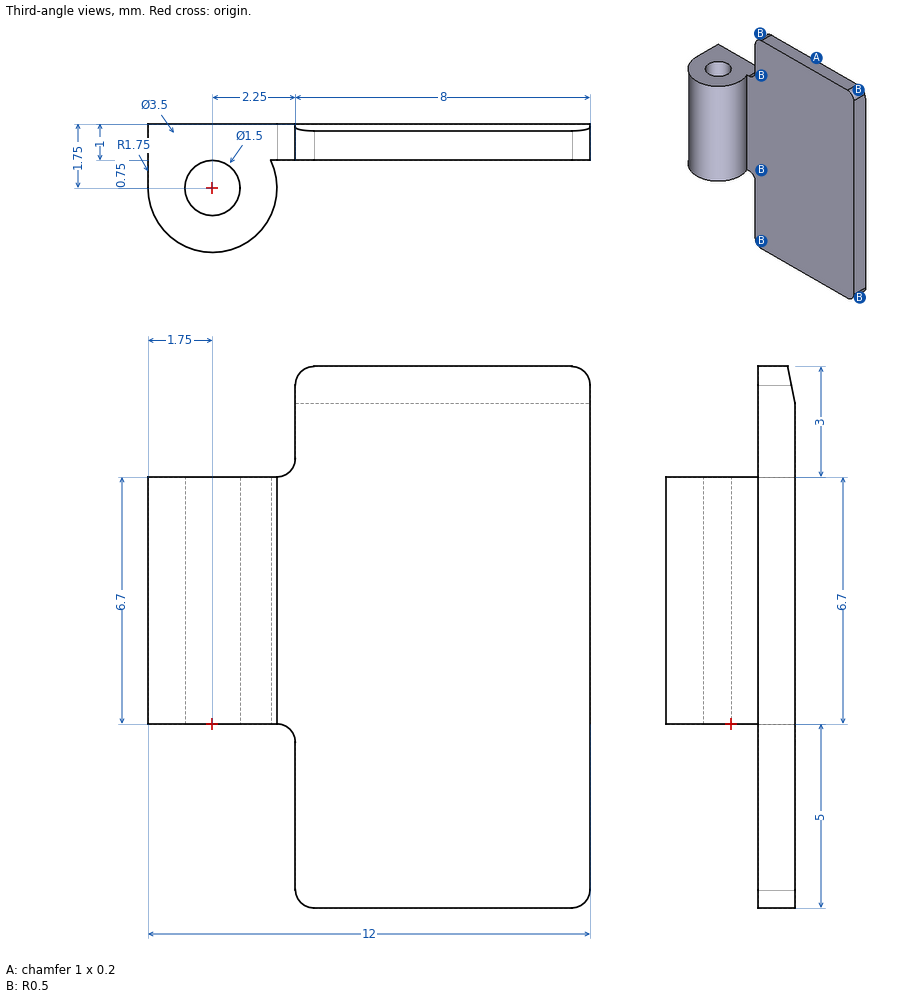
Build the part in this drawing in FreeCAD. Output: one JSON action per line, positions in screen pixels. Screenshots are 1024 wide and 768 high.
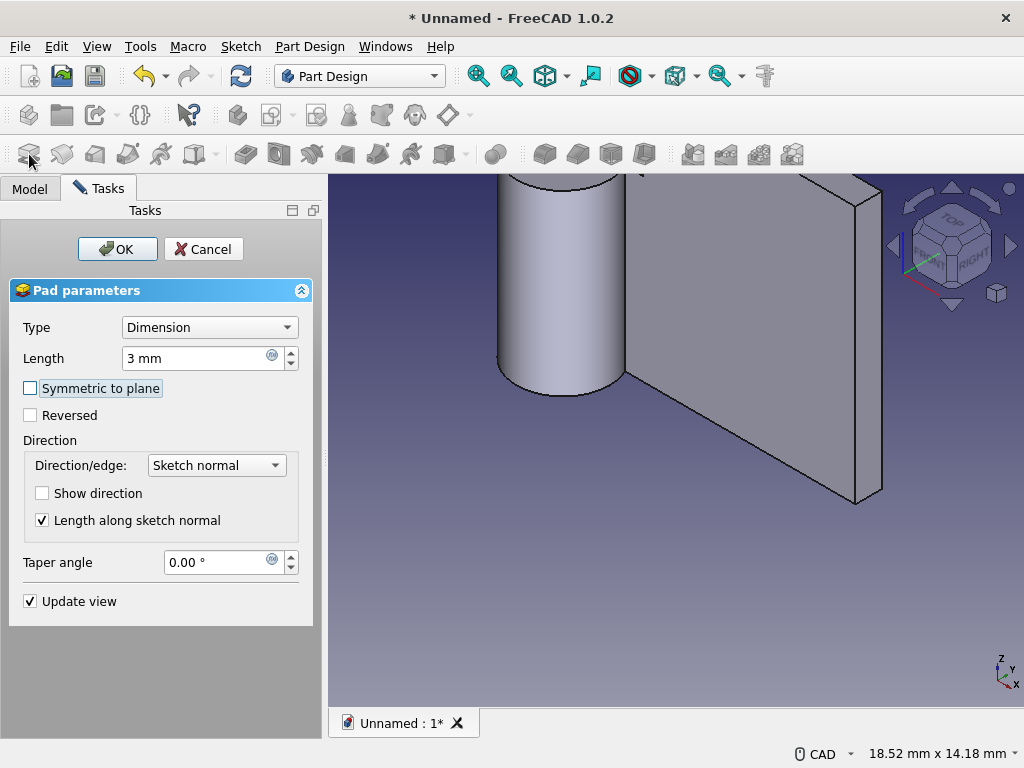
{"action": "left_click", "coordinate": [118, 249]}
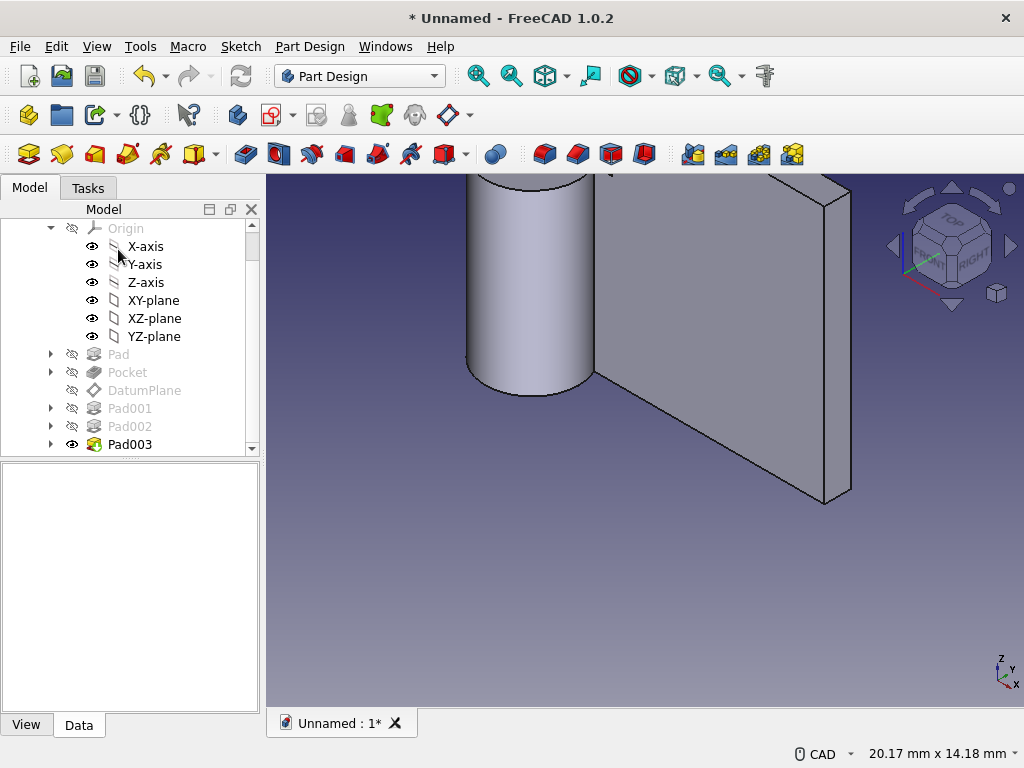
{"action": "left_click", "coordinate": [479, 76]}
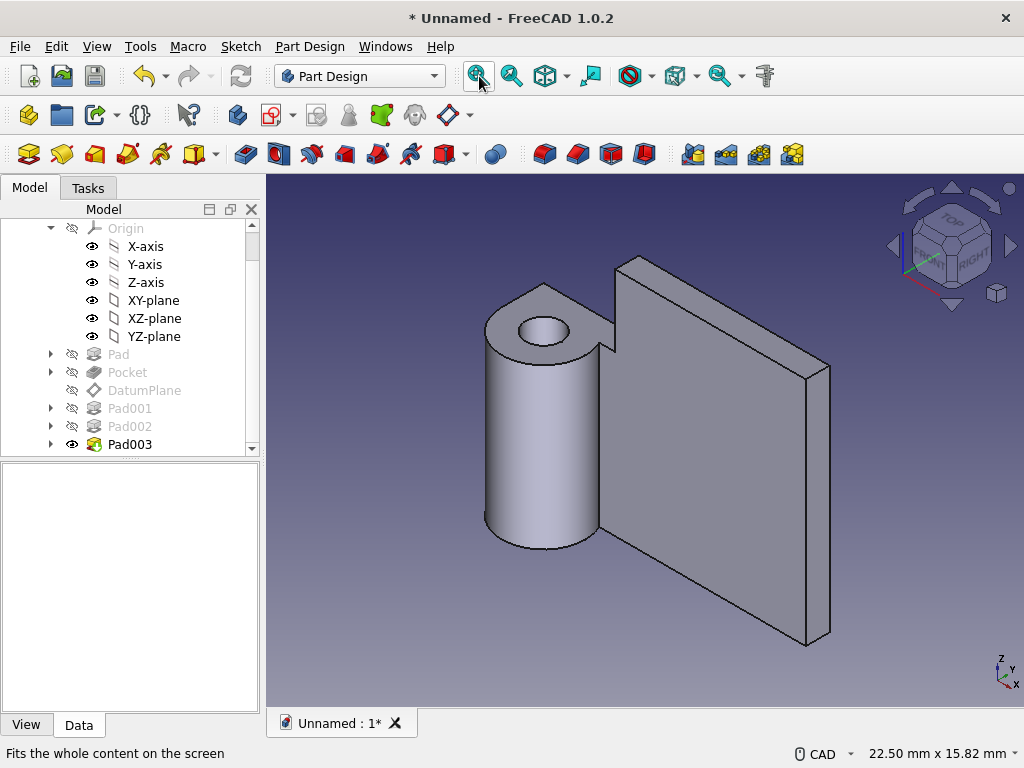
{"action": "key", "text": "5"}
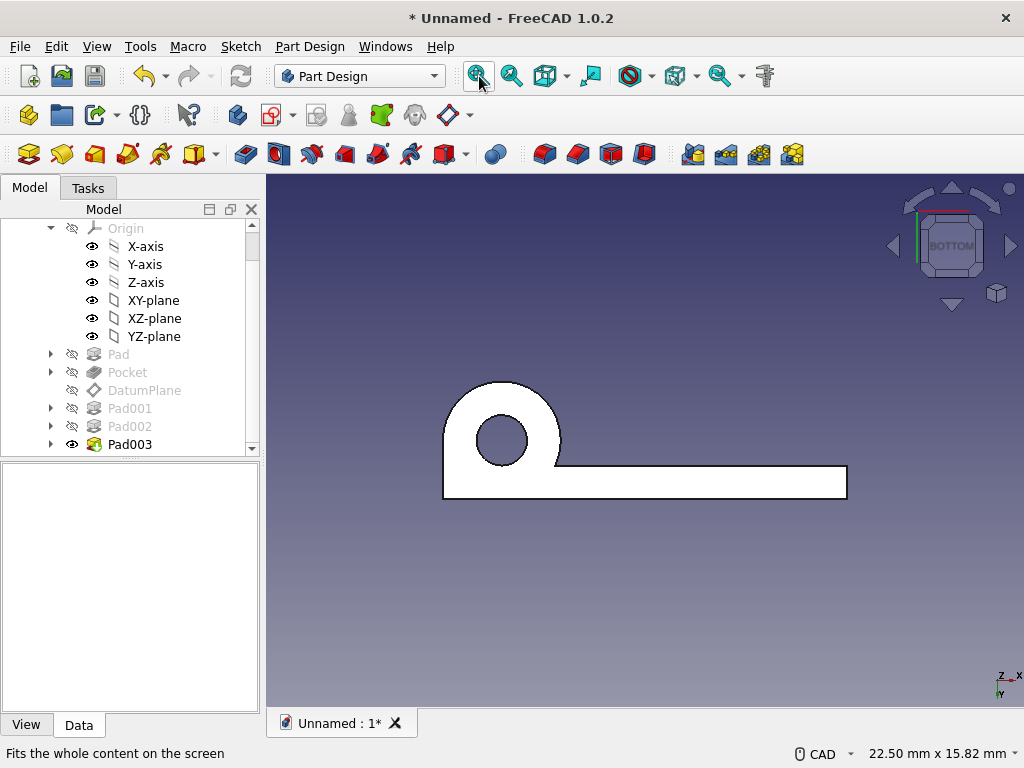
{"action": "left_click", "coordinate": [472, 473]}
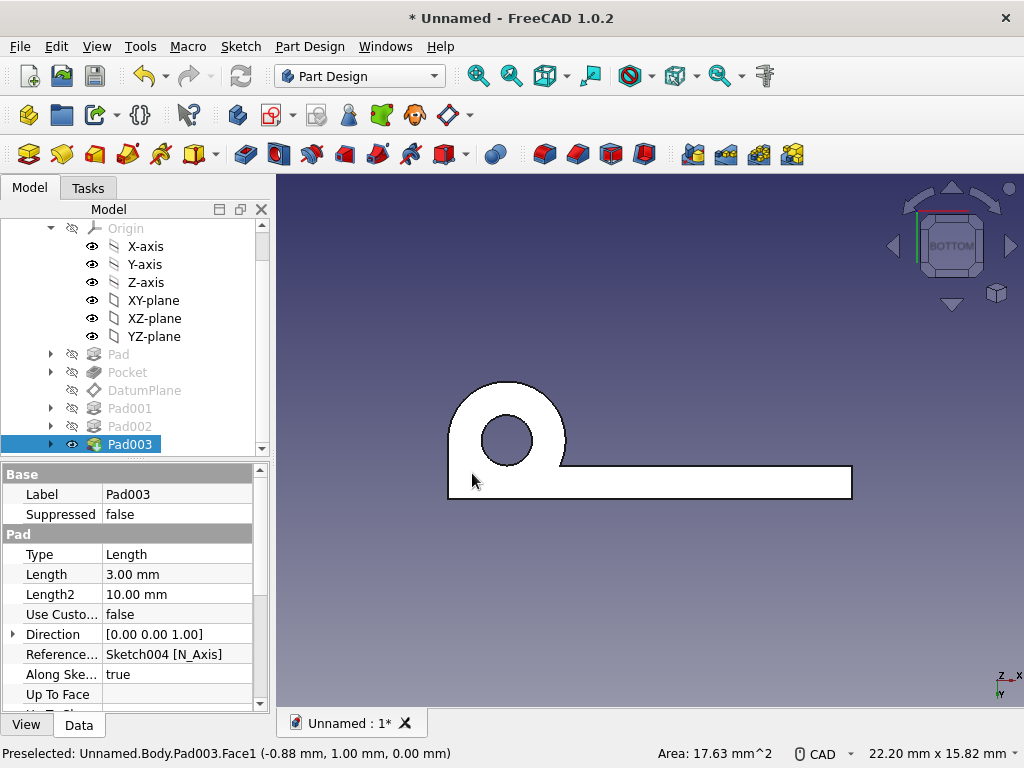
{"action": "left_click", "coordinate": [270, 116]}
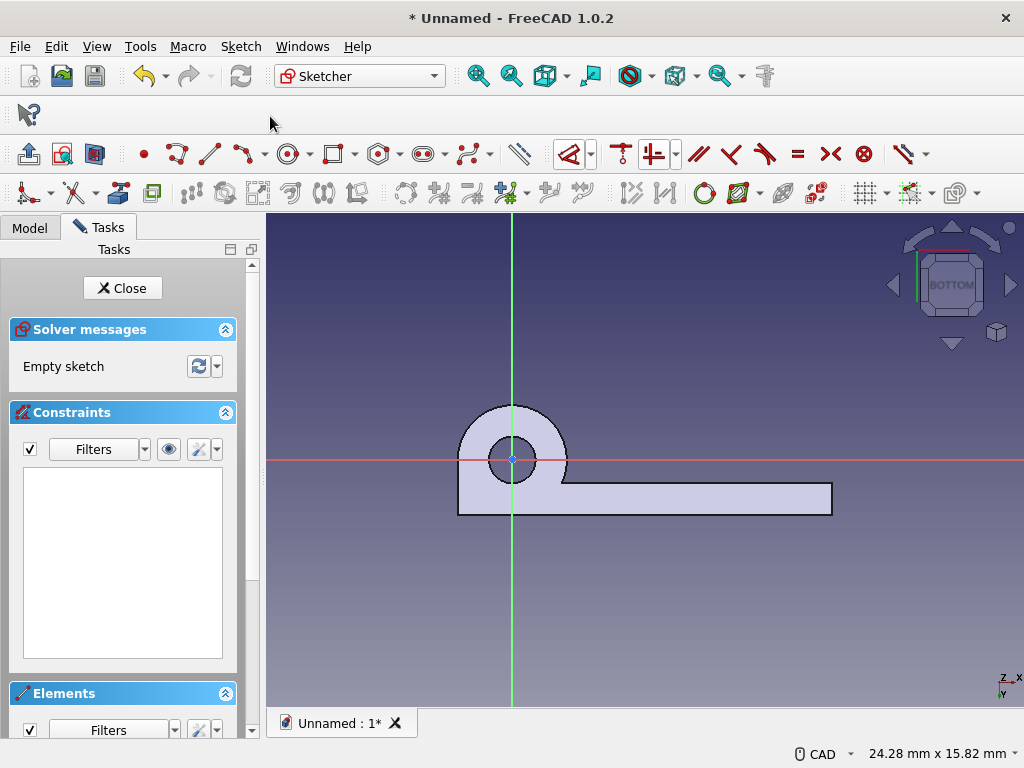
{"action": "left_click", "coordinate": [332, 154]}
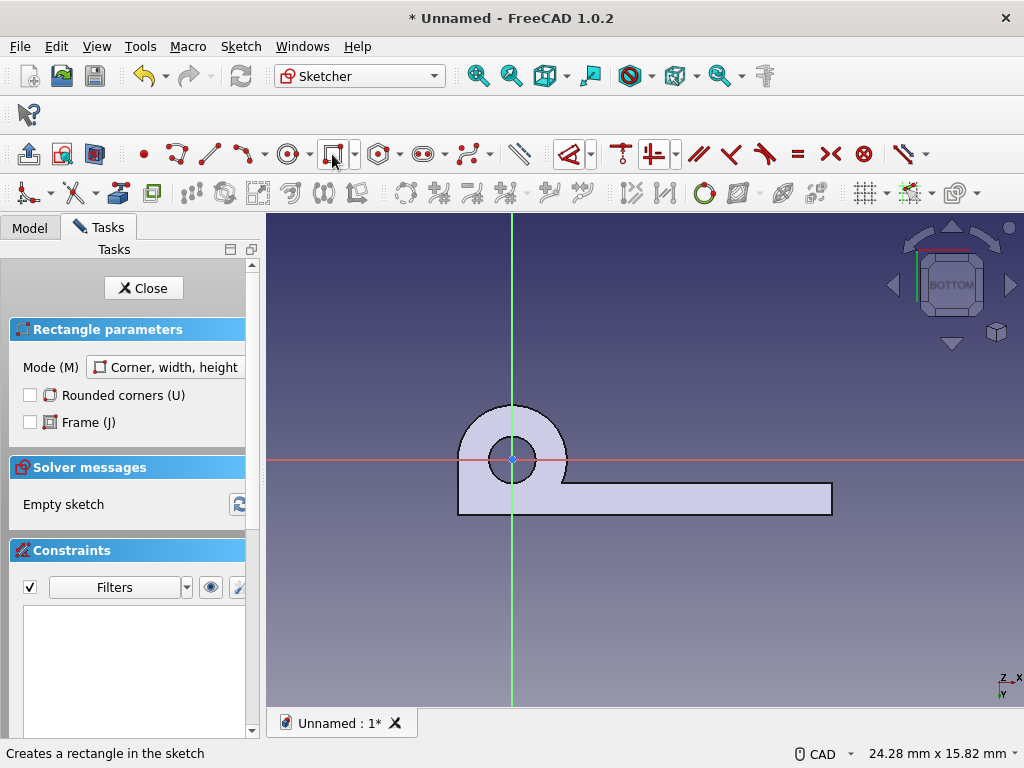
{"action": "left_click", "coordinate": [583, 483]}
{"action": "left_click", "coordinate": [832, 515]}
{"action": "key", "text": "Escape"}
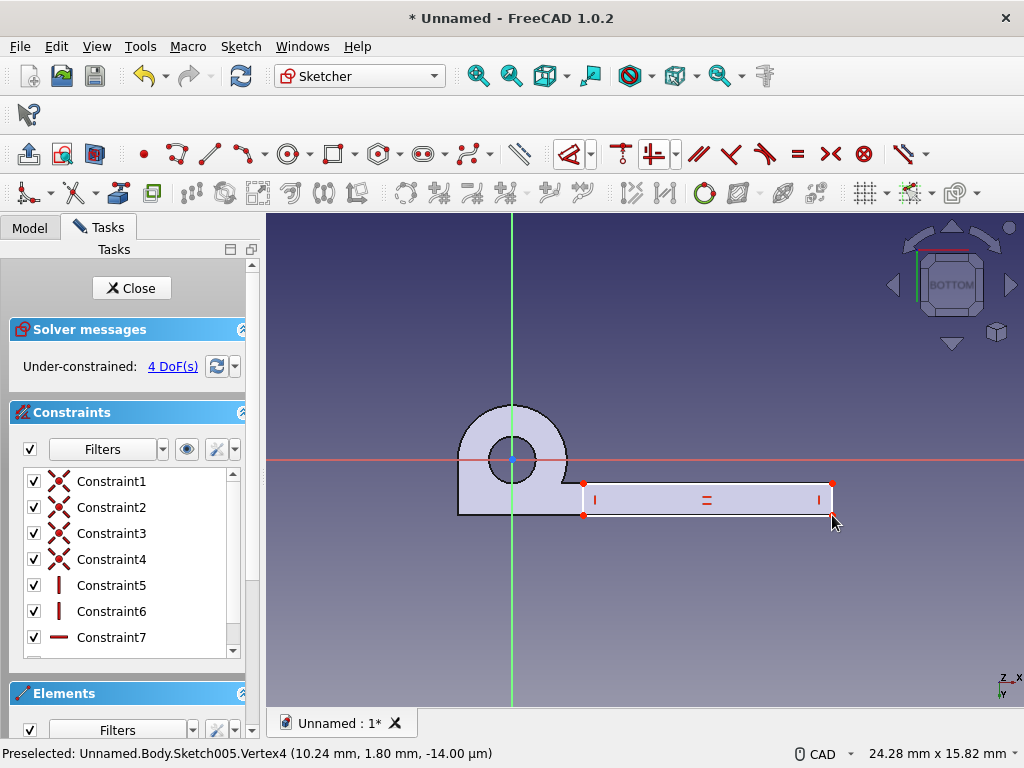
{"action": "scroll", "coordinate": [583, 494], "scroll_direction": "up", "scroll_amount": 2}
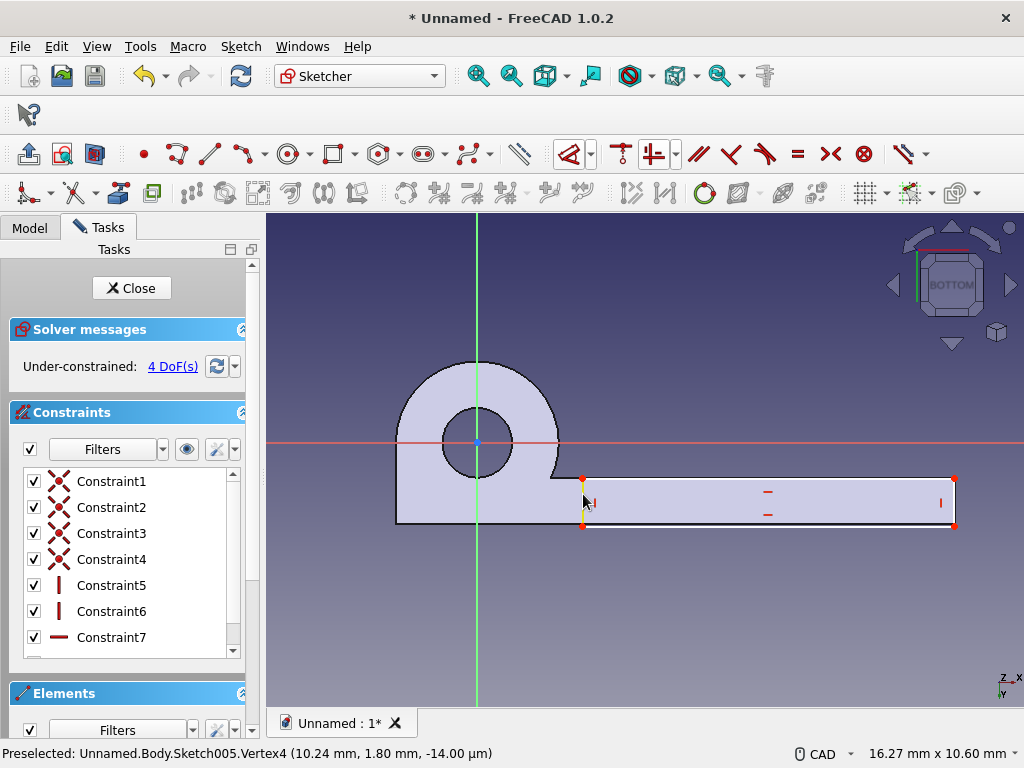
{"action": "left_click", "coordinate": [583, 493]}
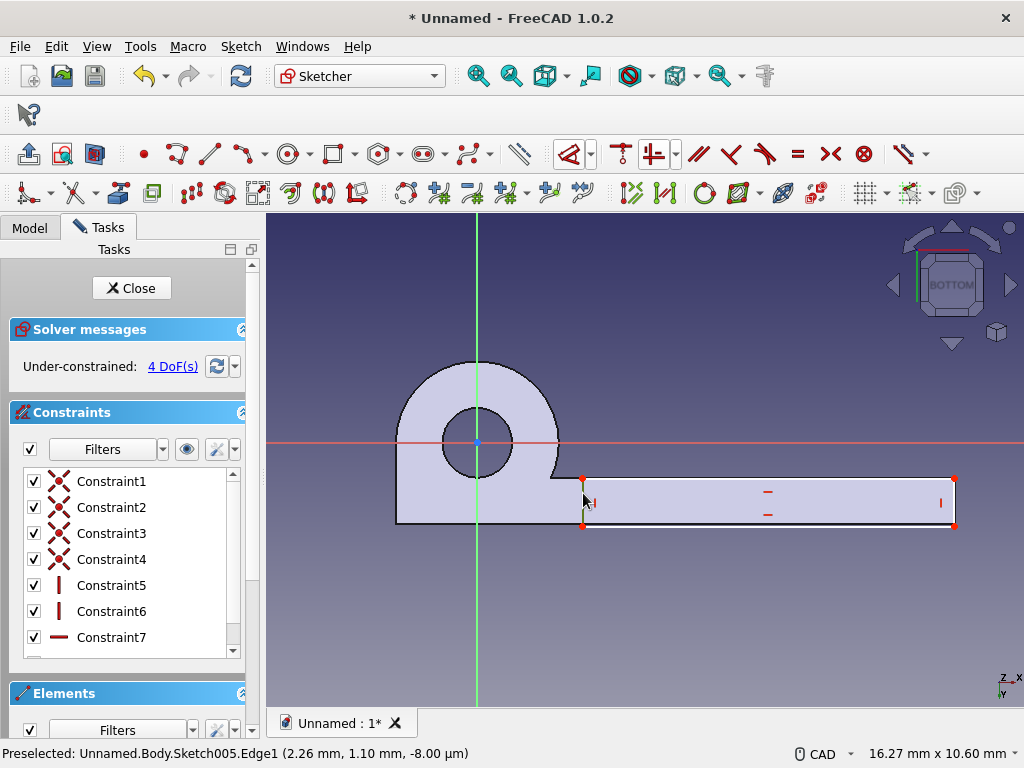
{"action": "key", "text": "i"}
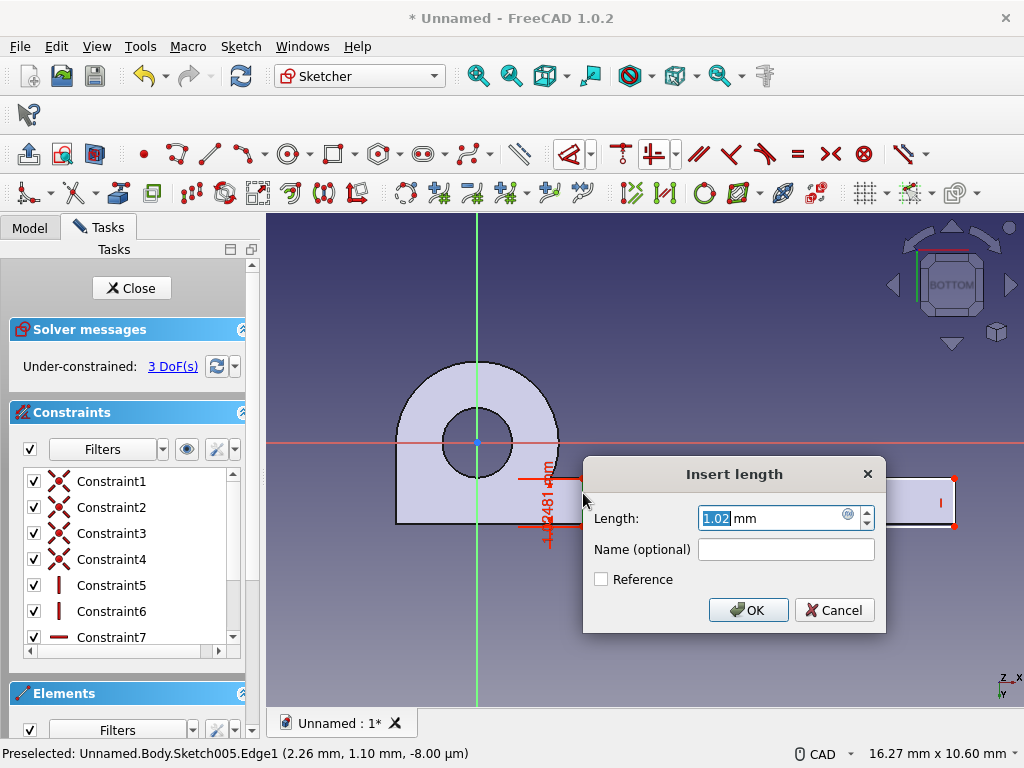
{"action": "type", "text": "1"}
{"action": "key", "text": "Return"}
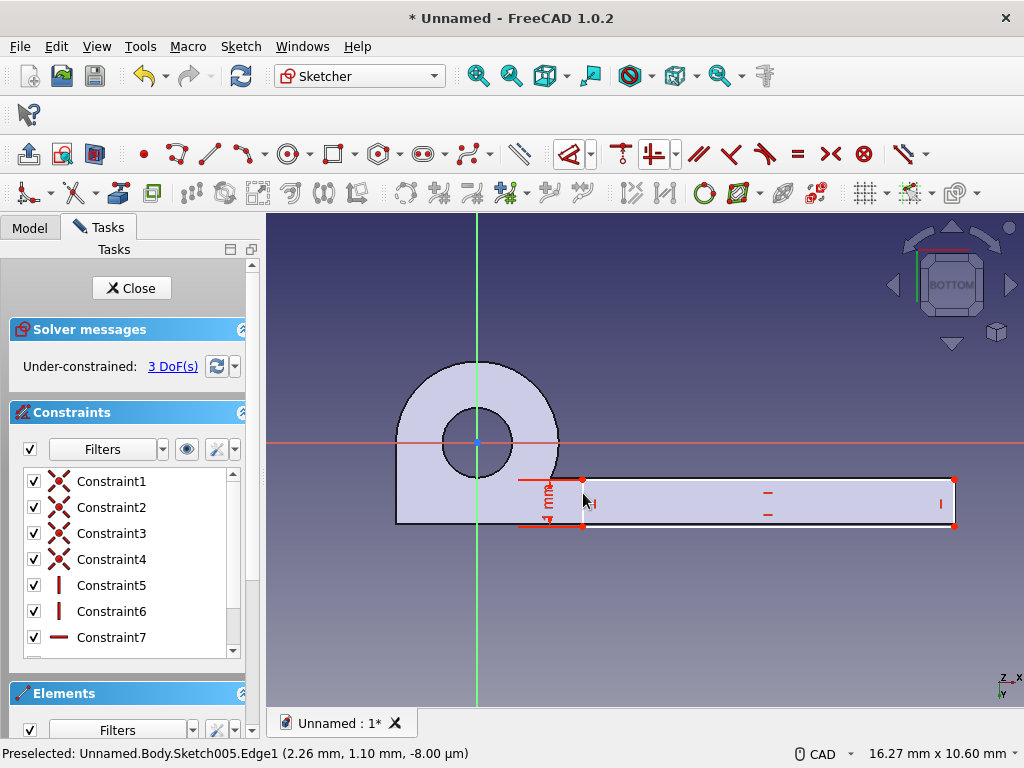
{"action": "left_click", "coordinate": [694, 527]}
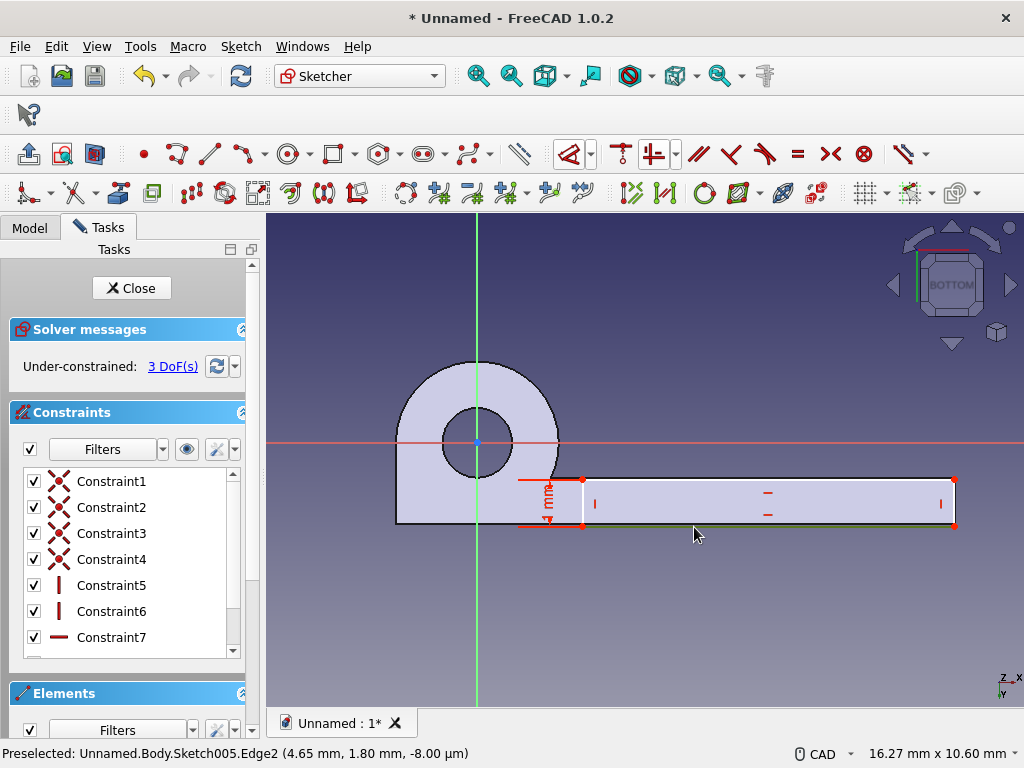
{"action": "left_click", "coordinate": [590, 154]}